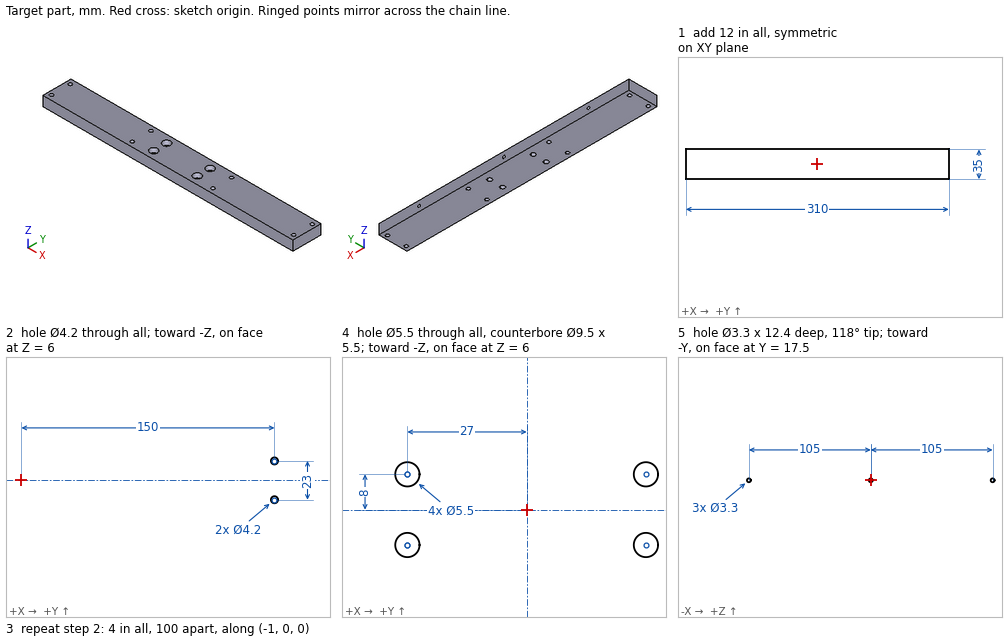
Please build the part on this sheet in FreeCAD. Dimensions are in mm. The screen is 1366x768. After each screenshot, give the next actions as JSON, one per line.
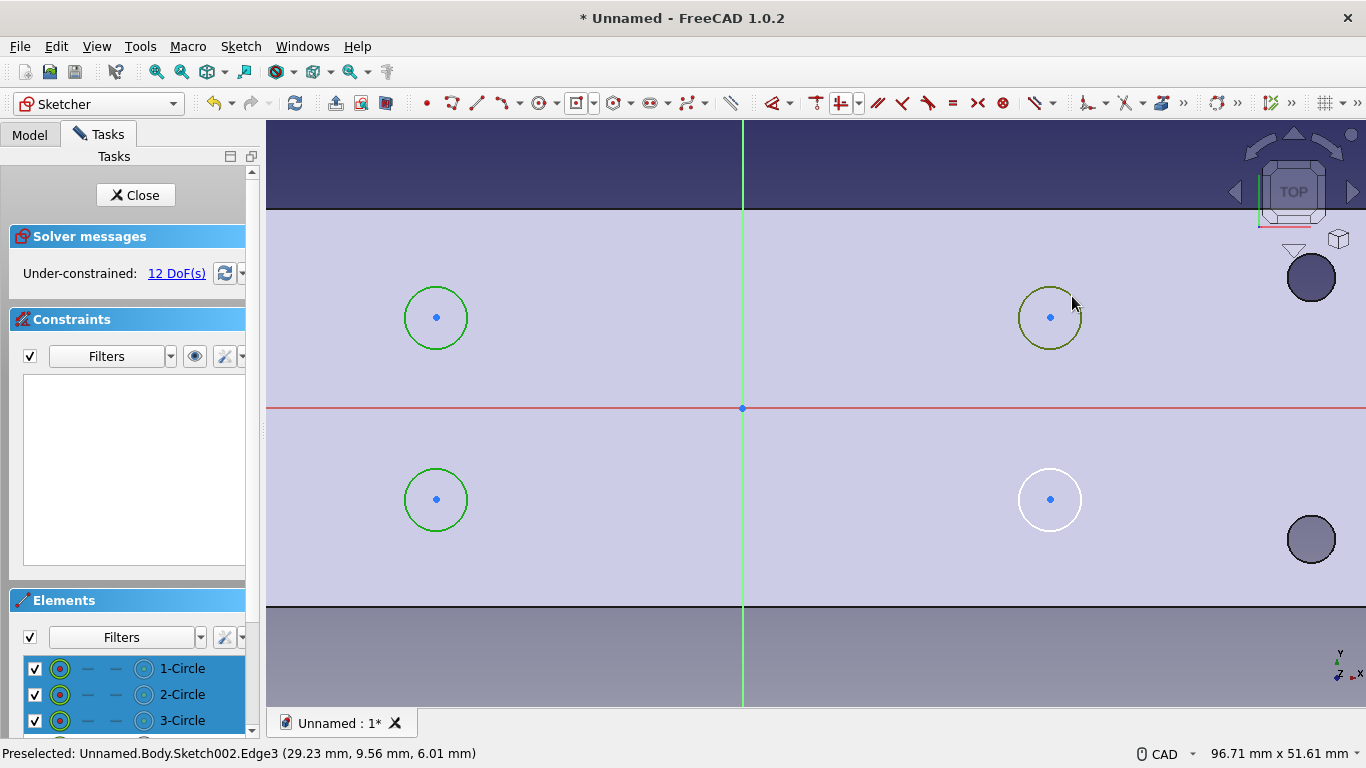
{"action": "left_click", "coordinate": [1072, 478]}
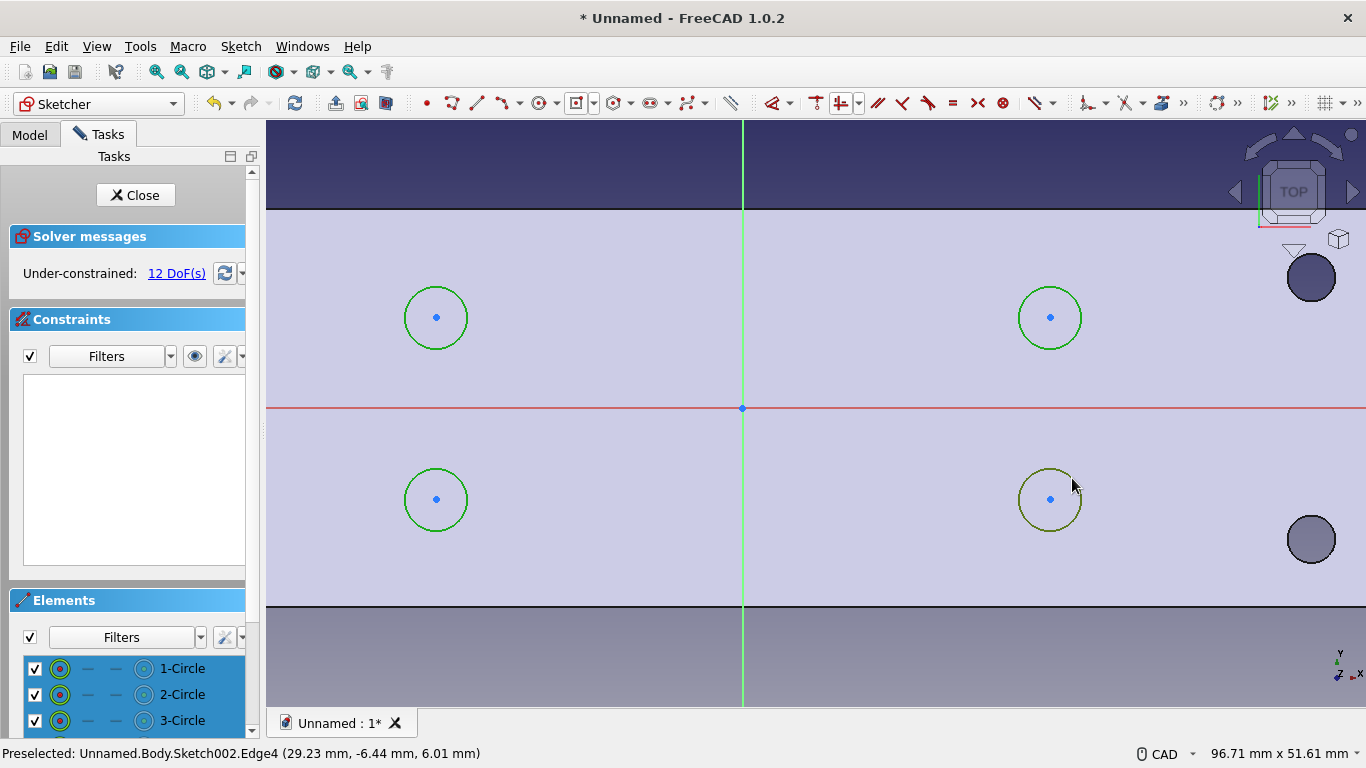
{"action": "left_click", "coordinate": [953, 104]}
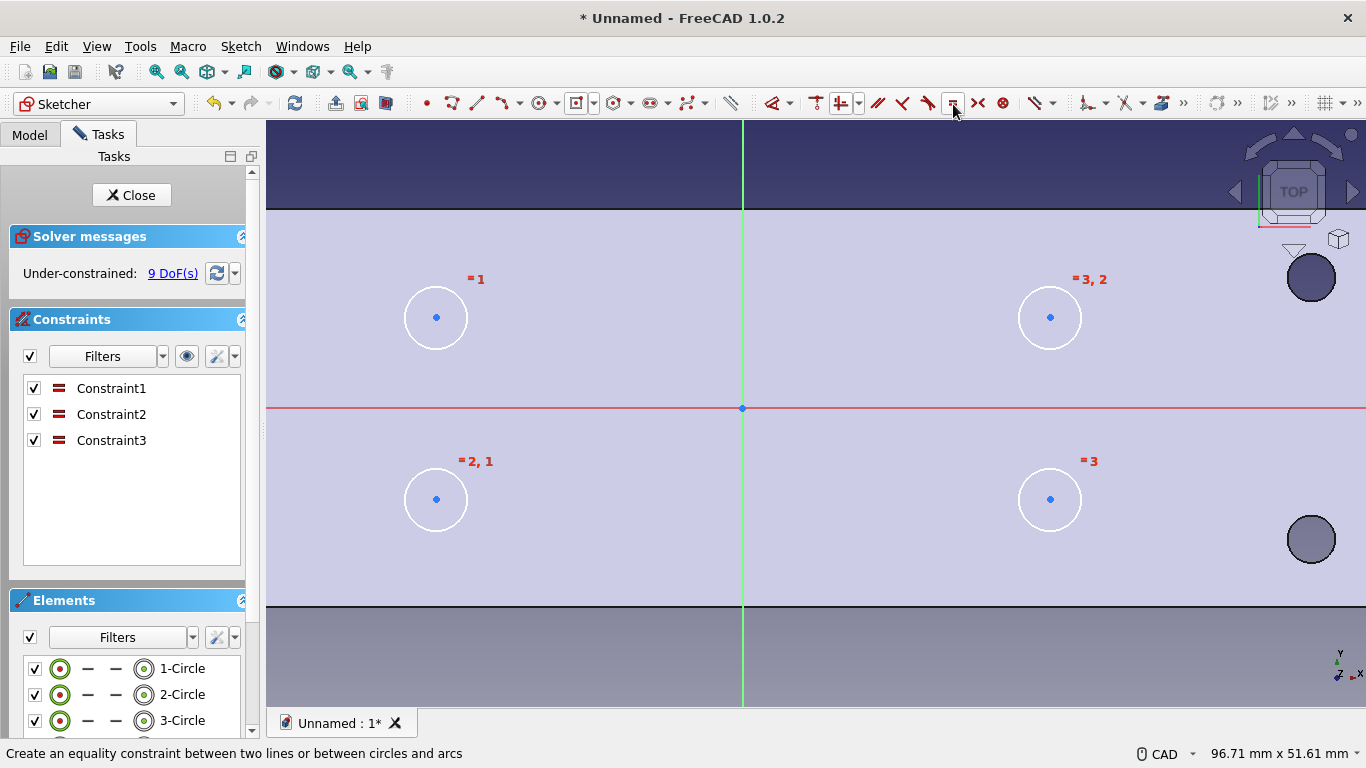
{"action": "left_click", "coordinate": [436, 318]}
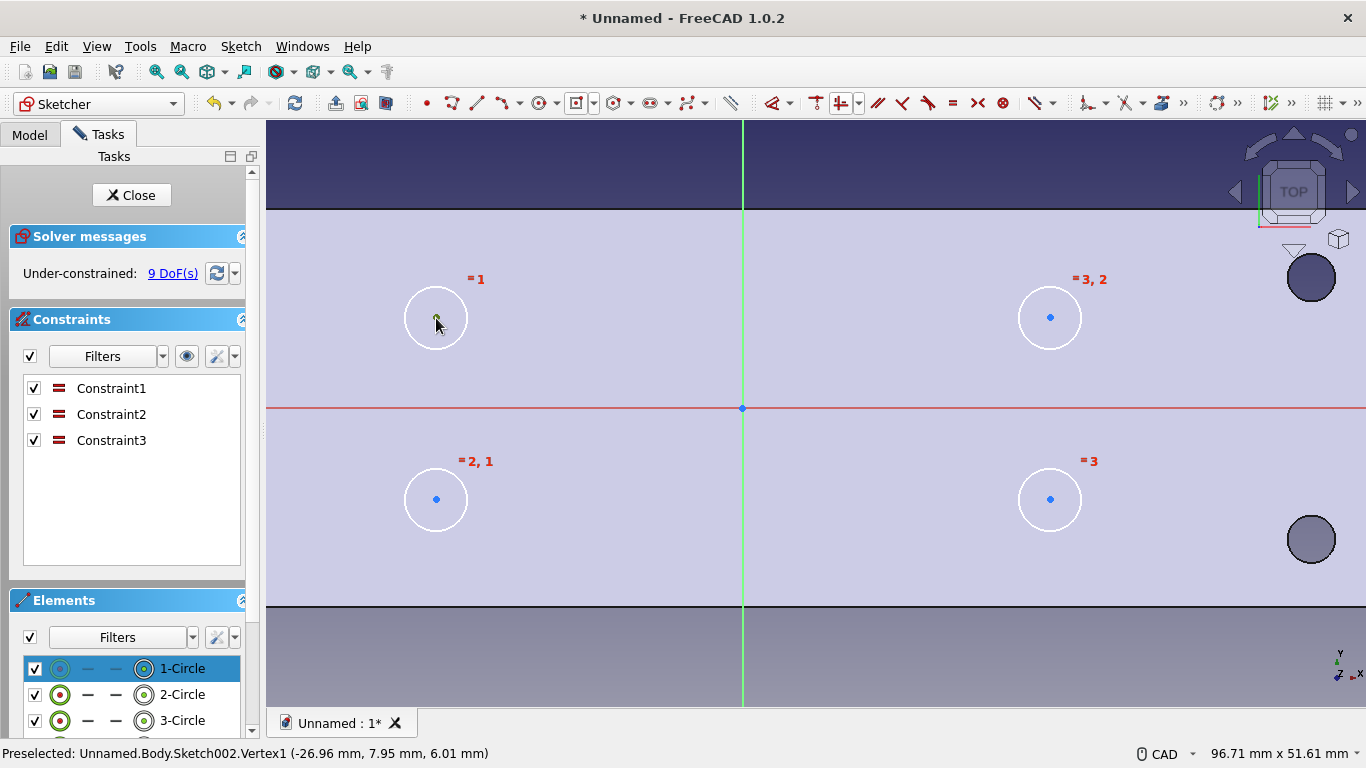
{"action": "left_click", "coordinate": [436, 500]}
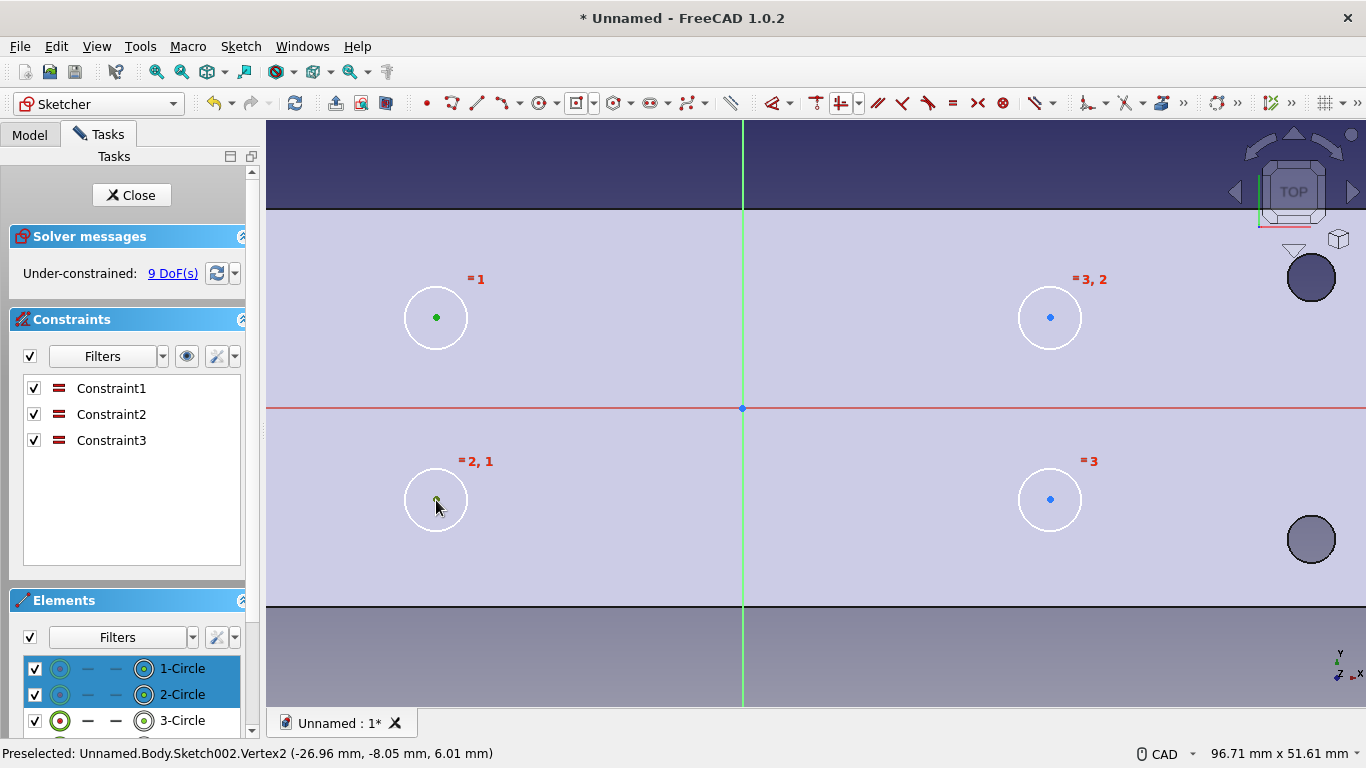
{"action": "left_click", "coordinate": [359, 408]}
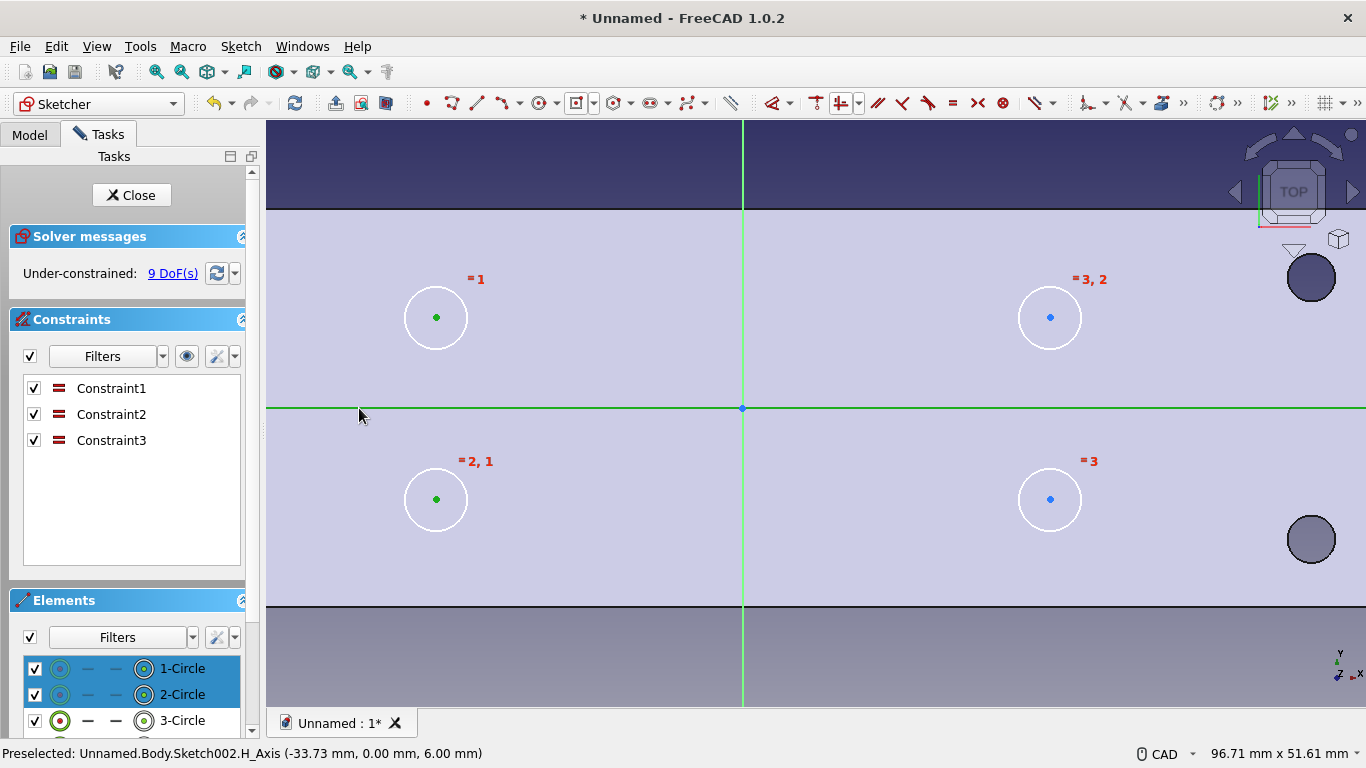
{"action": "left_click", "coordinate": [978, 104]}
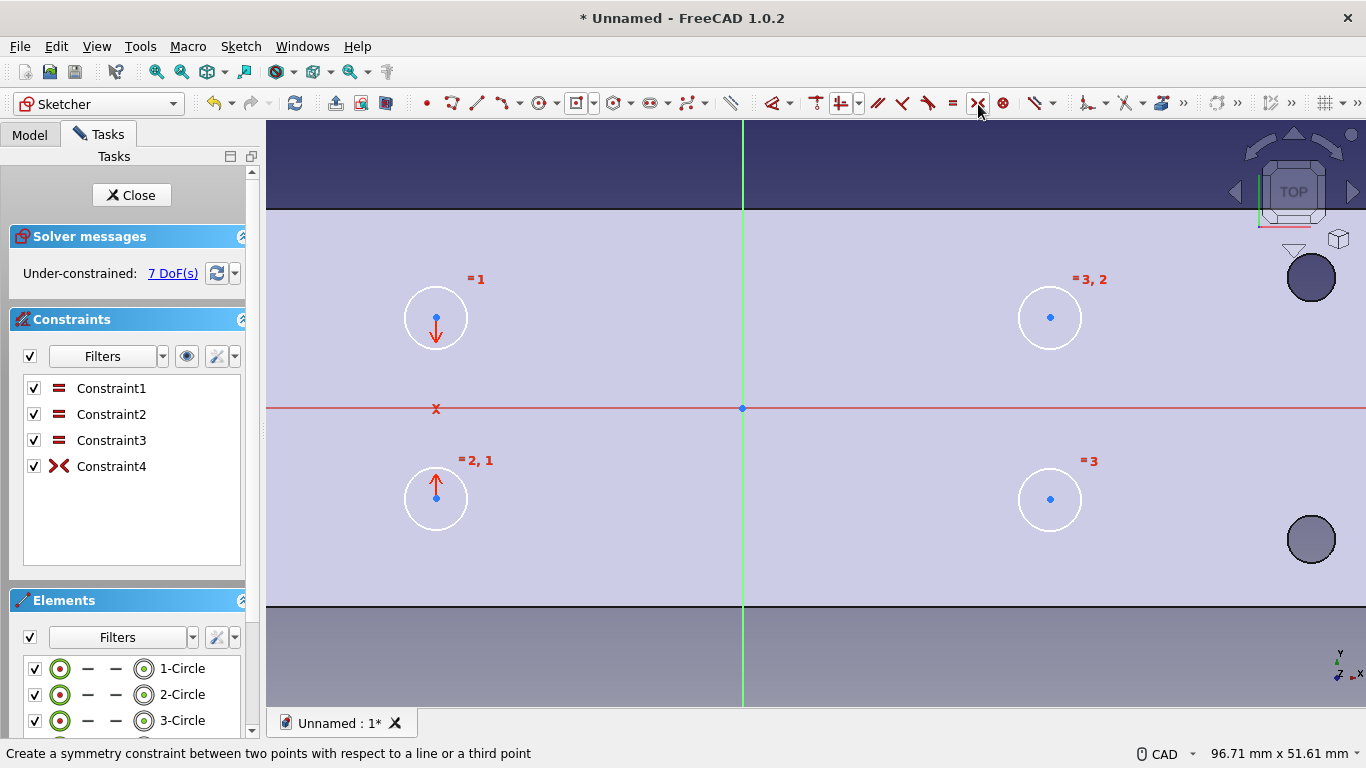
{"action": "left_click", "coordinate": [436, 318]}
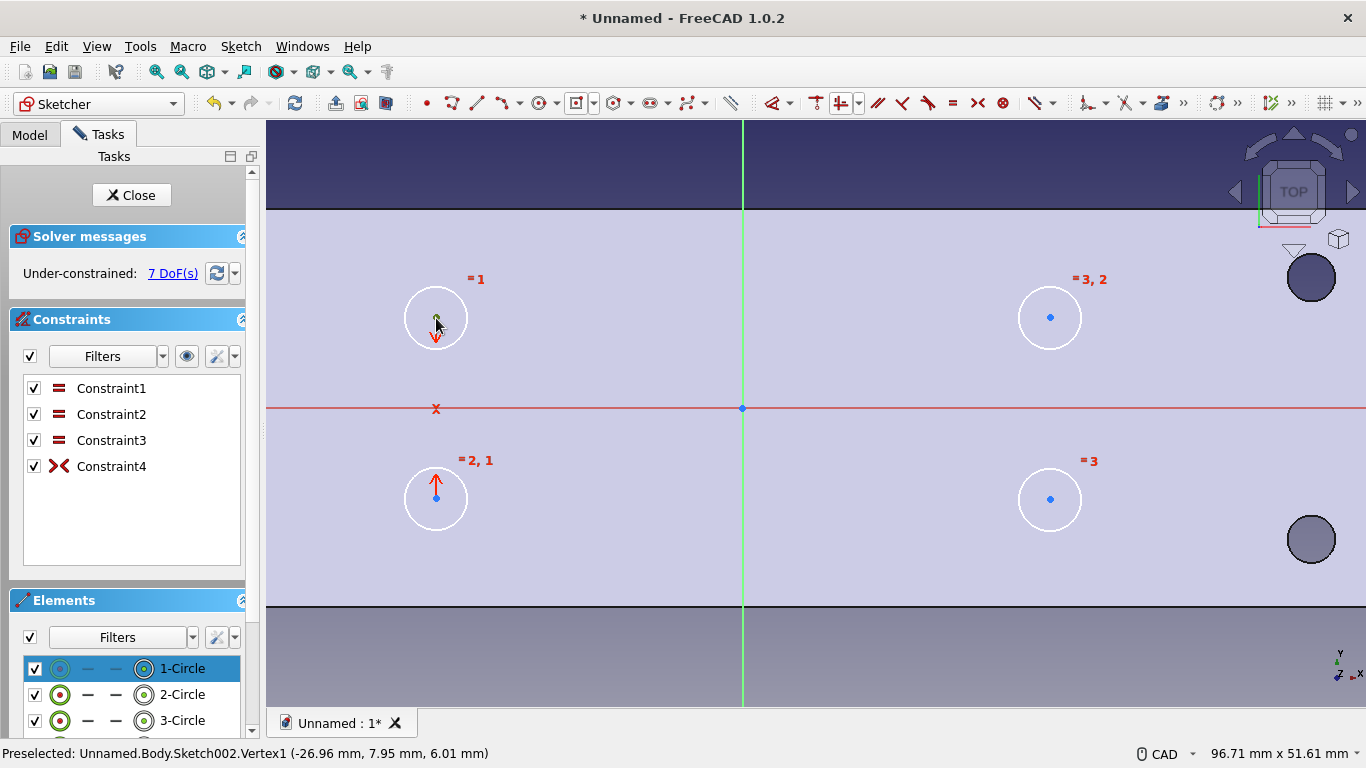
{"action": "left_click", "coordinate": [1050, 318]}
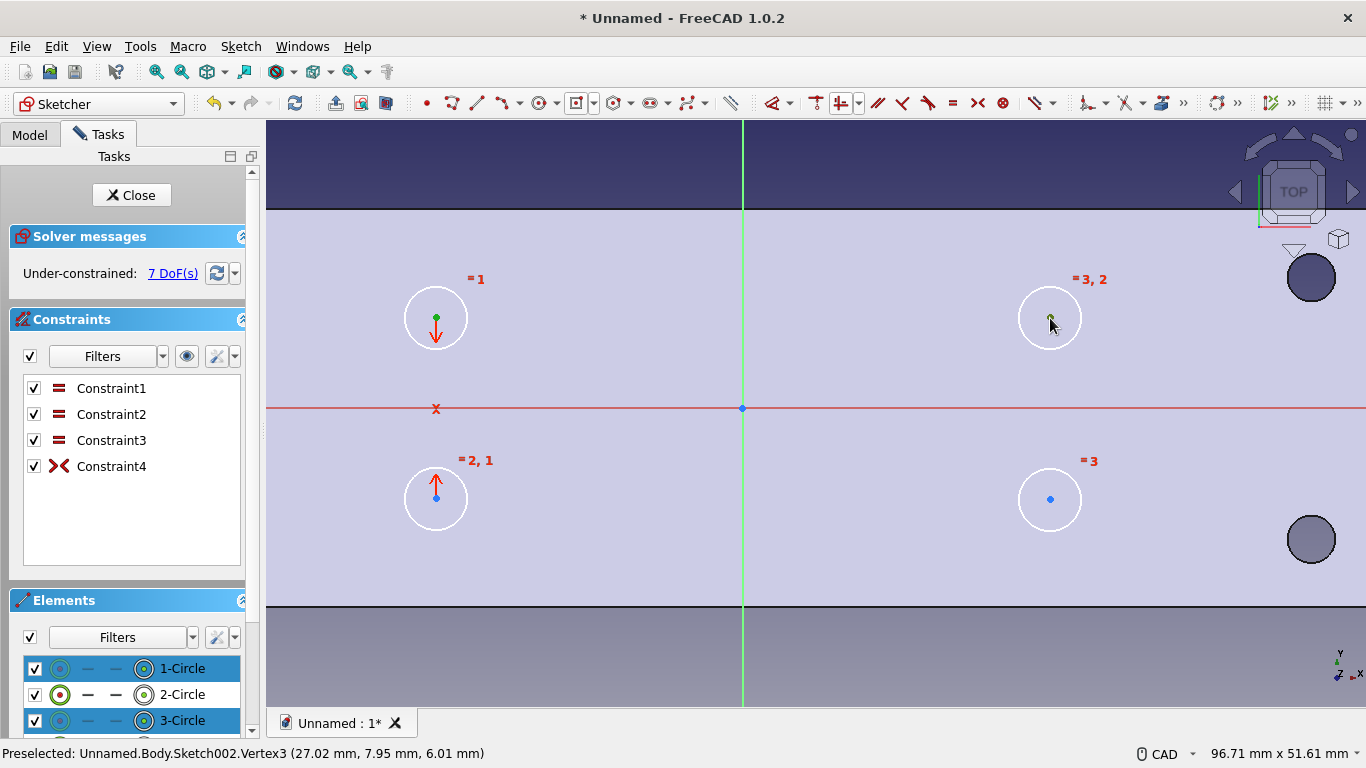
{"action": "left_click", "coordinate": [743, 641]}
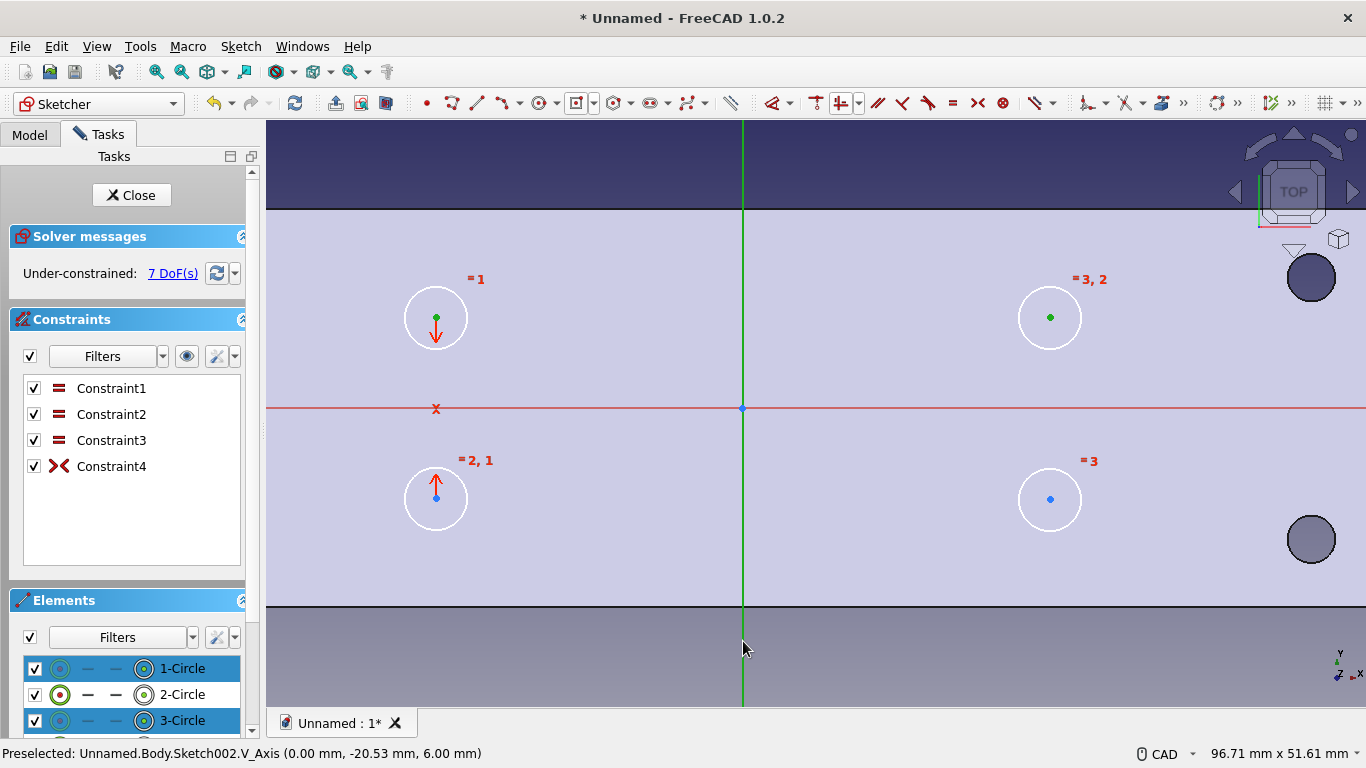
{"action": "left_click", "coordinate": [978, 104]}